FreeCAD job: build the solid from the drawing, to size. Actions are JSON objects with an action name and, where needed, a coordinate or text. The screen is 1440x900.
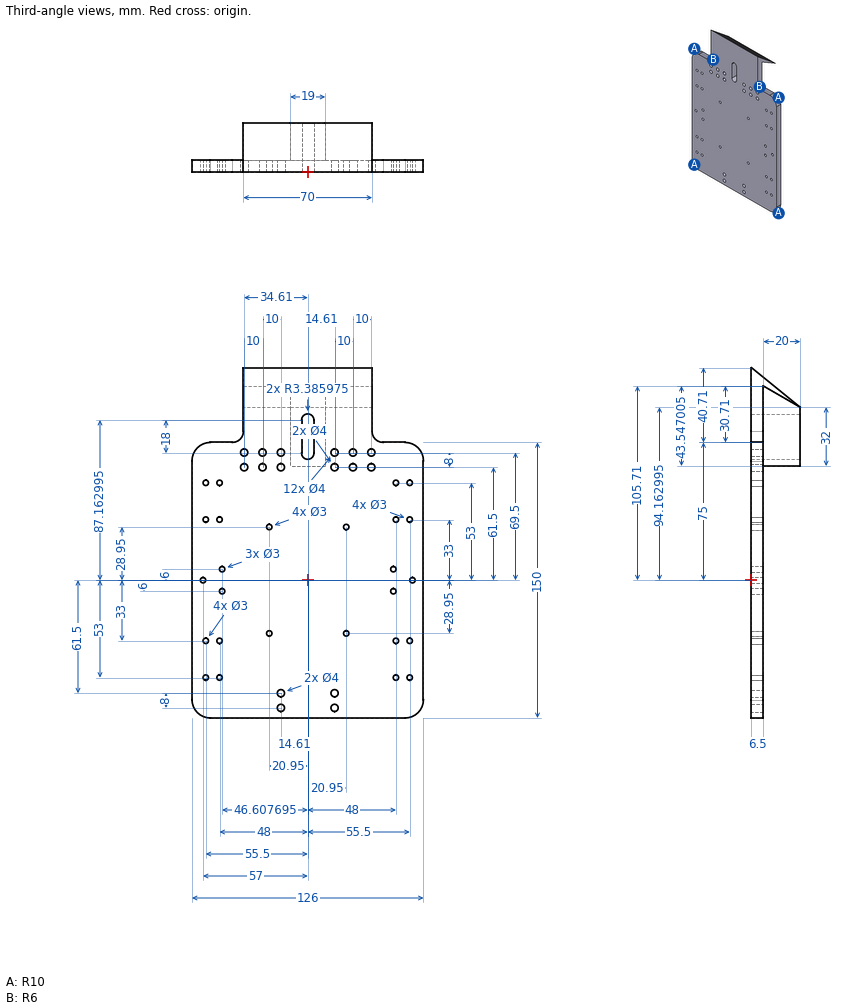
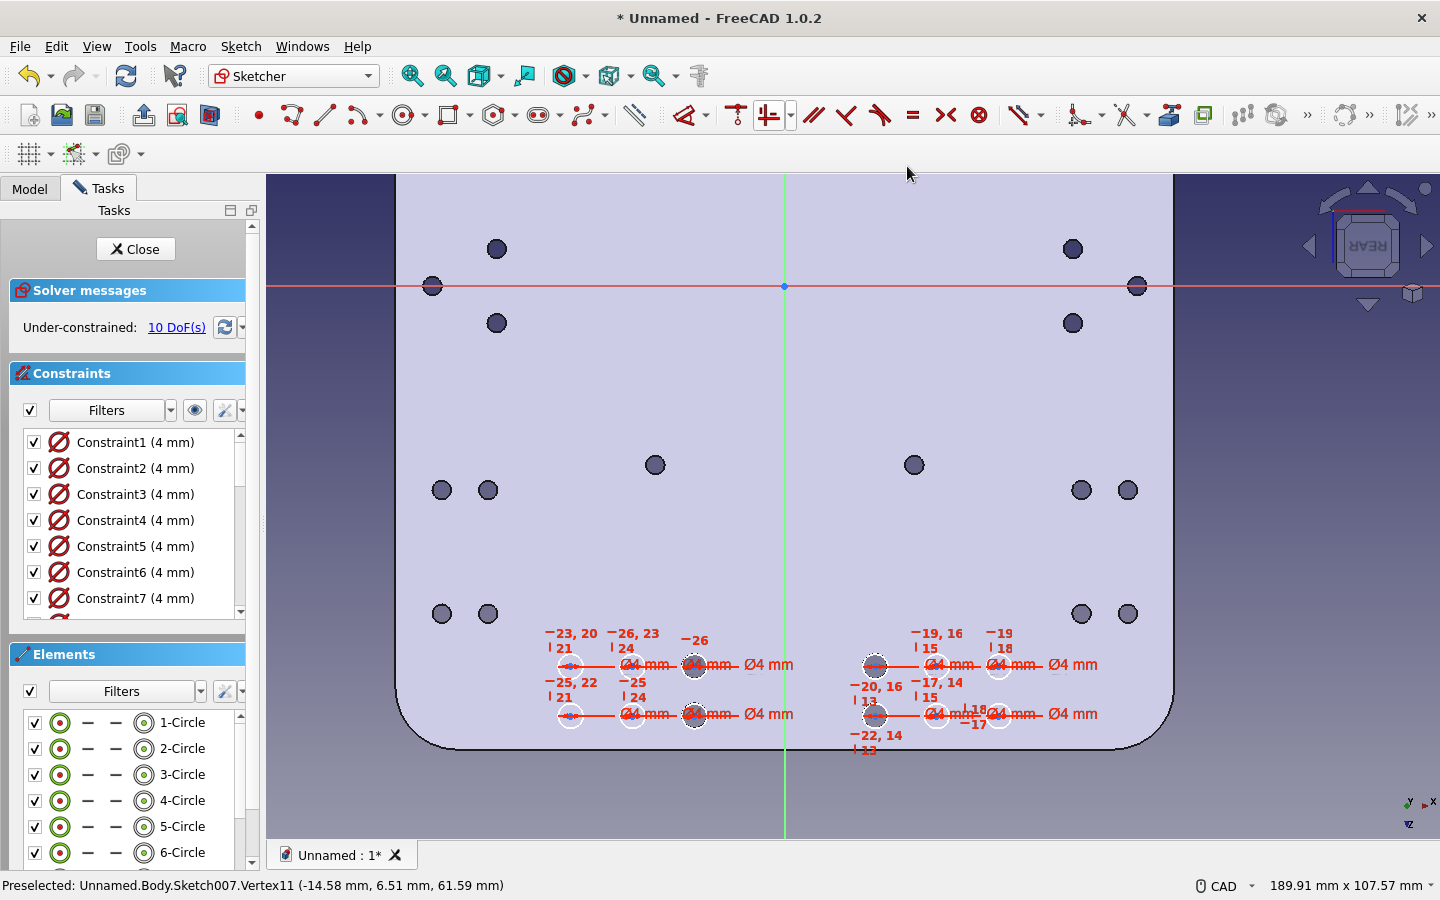
{"action": "left_click", "coordinate": [695, 667]}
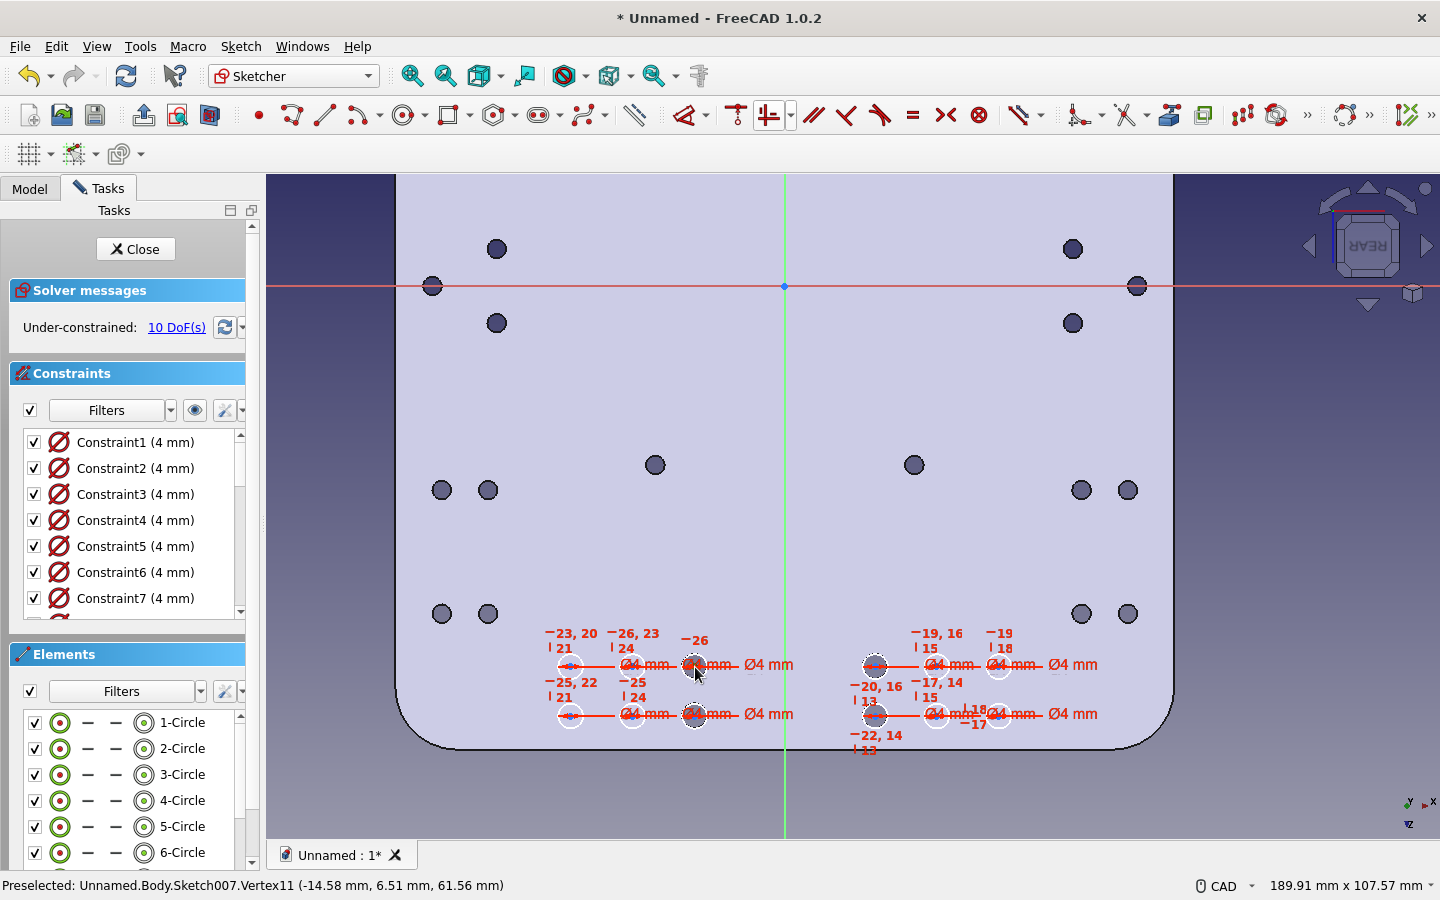
{"action": "left_click", "coordinate": [695, 716]}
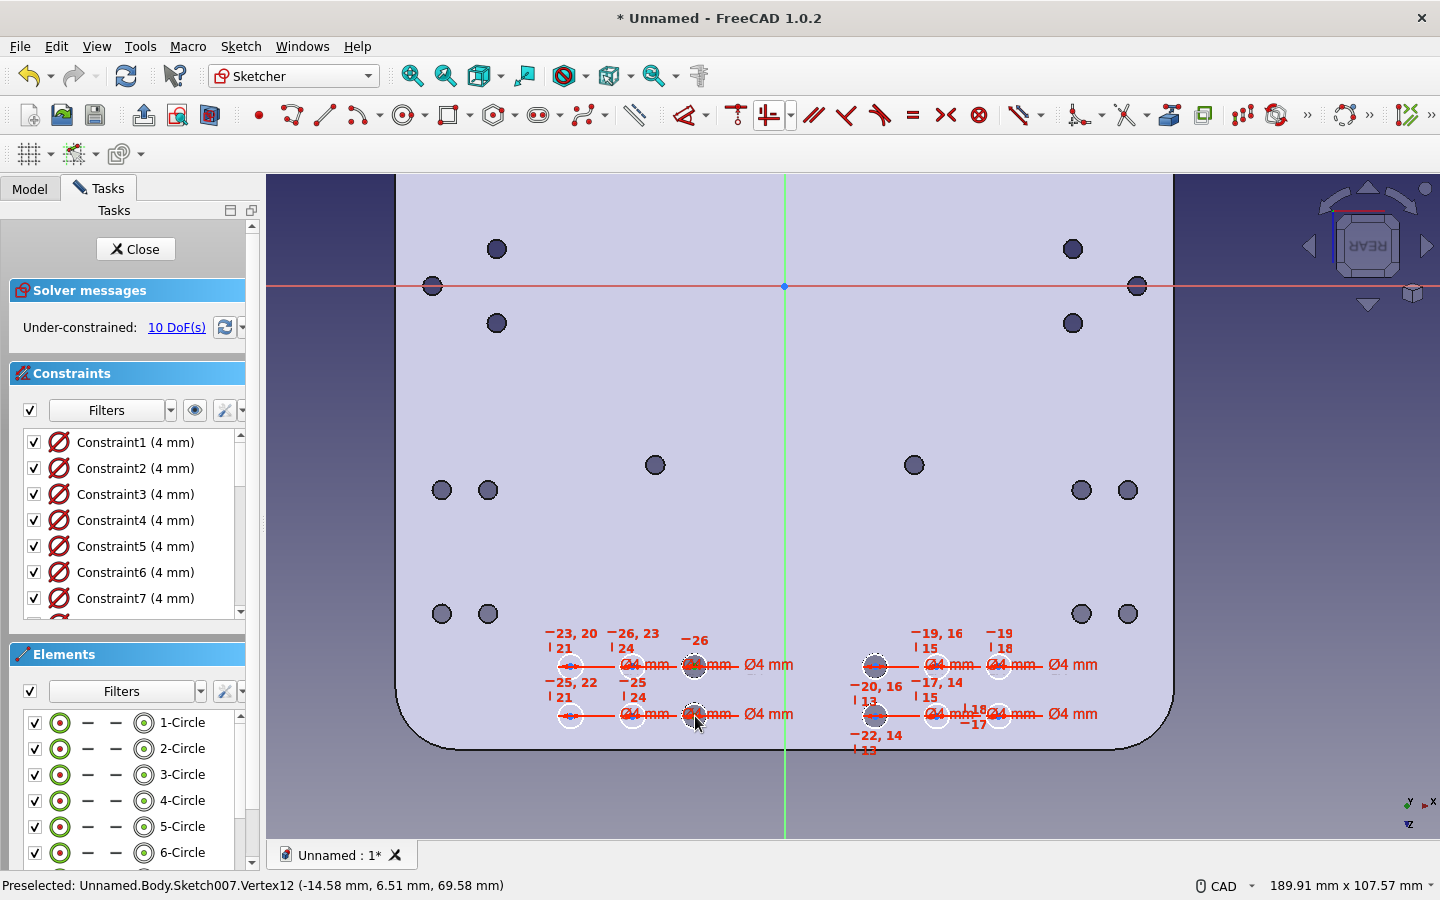
{"action": "key", "text": "v"}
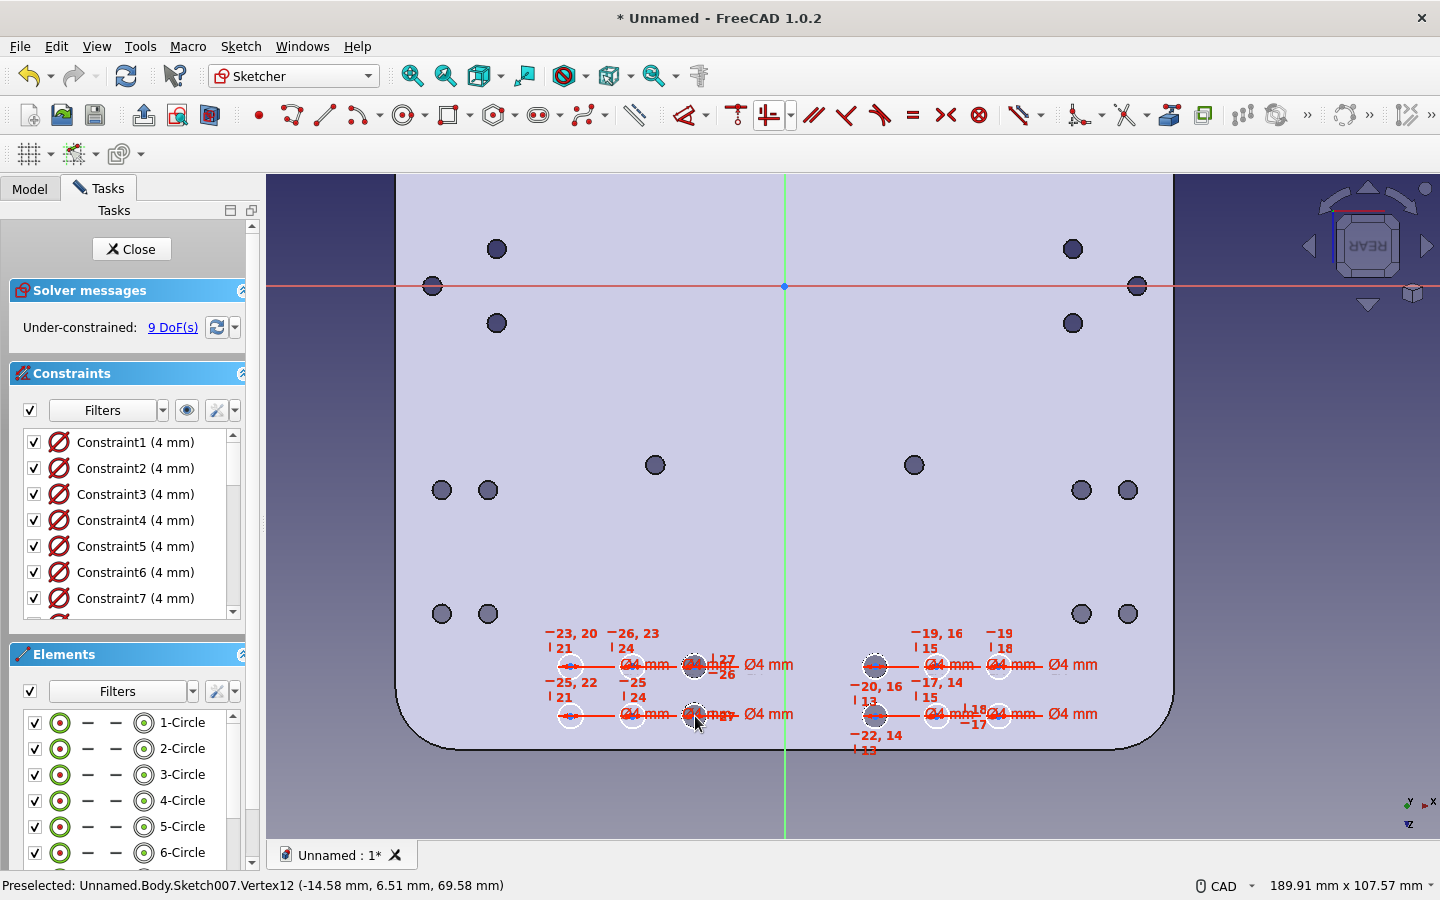
{"action": "left_click", "coordinate": [633, 716]}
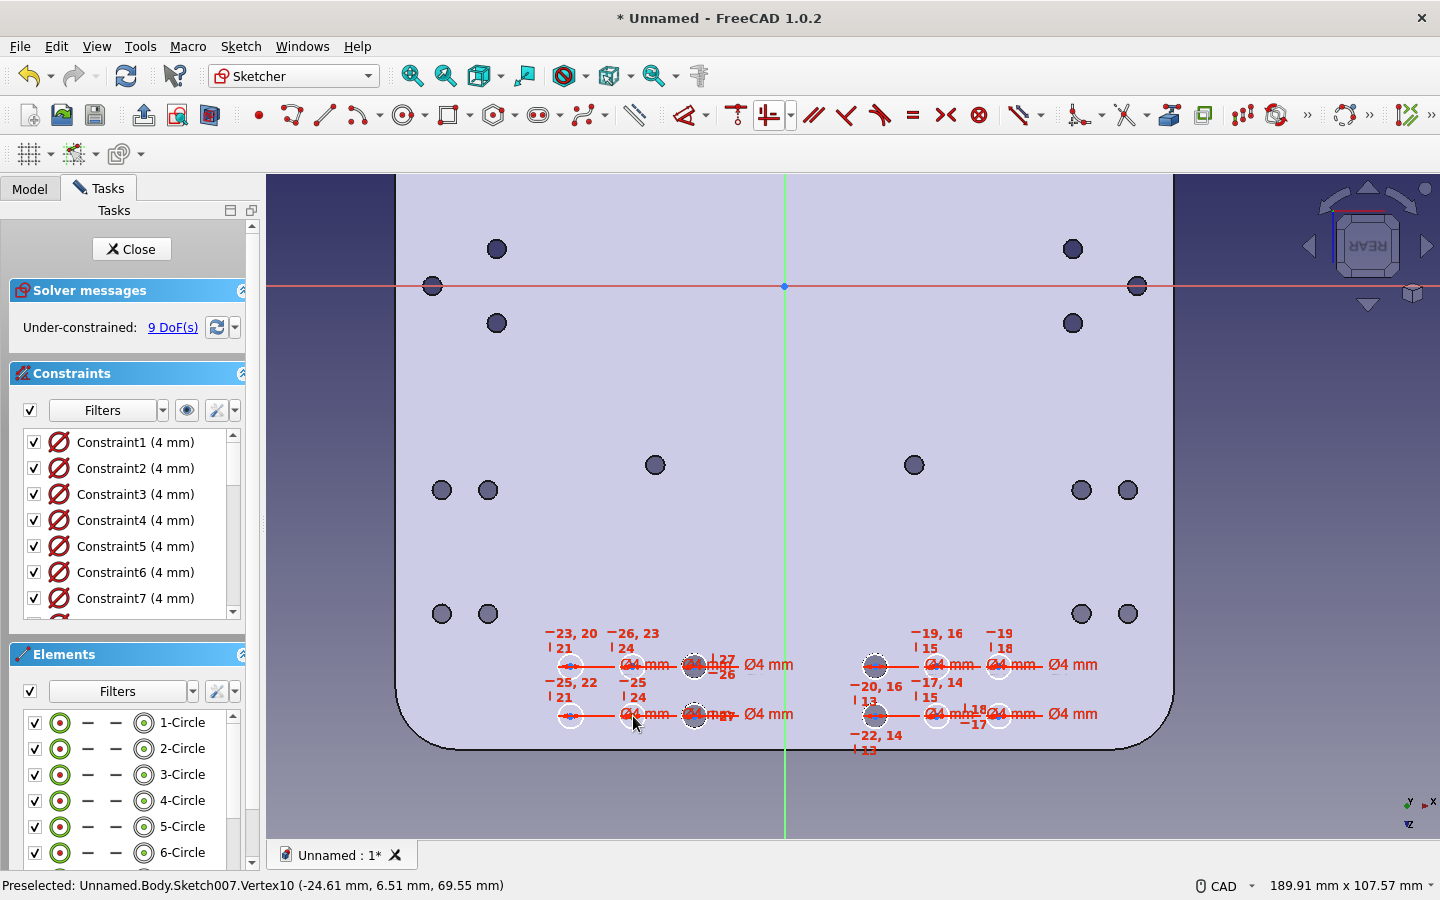
{"action": "left_click", "coordinate": [695, 716]}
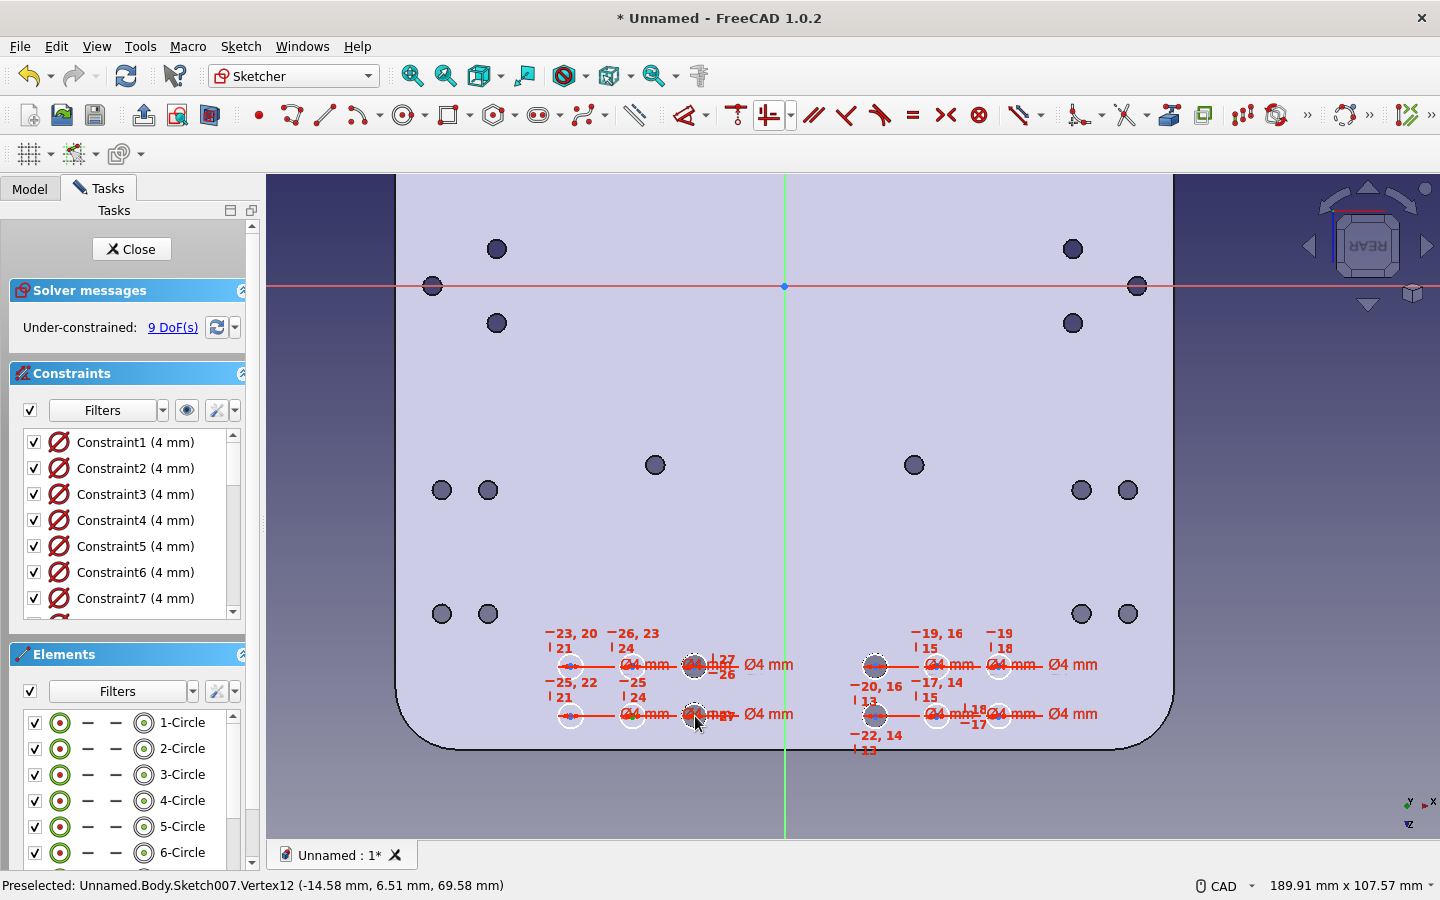
{"action": "key", "text": "h"}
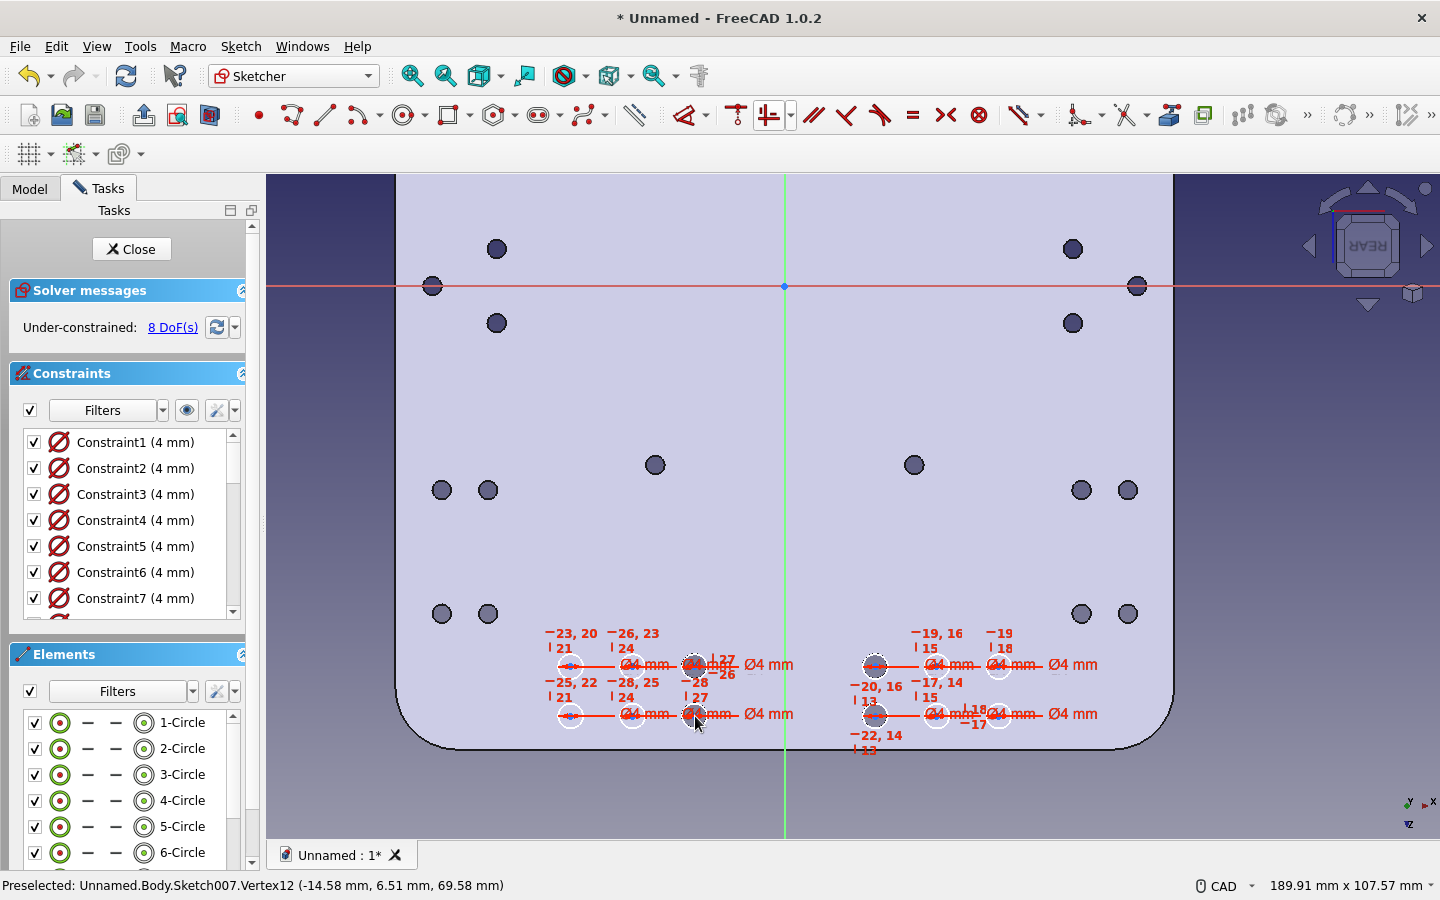
{"action": "left_click", "coordinate": [684, 116]}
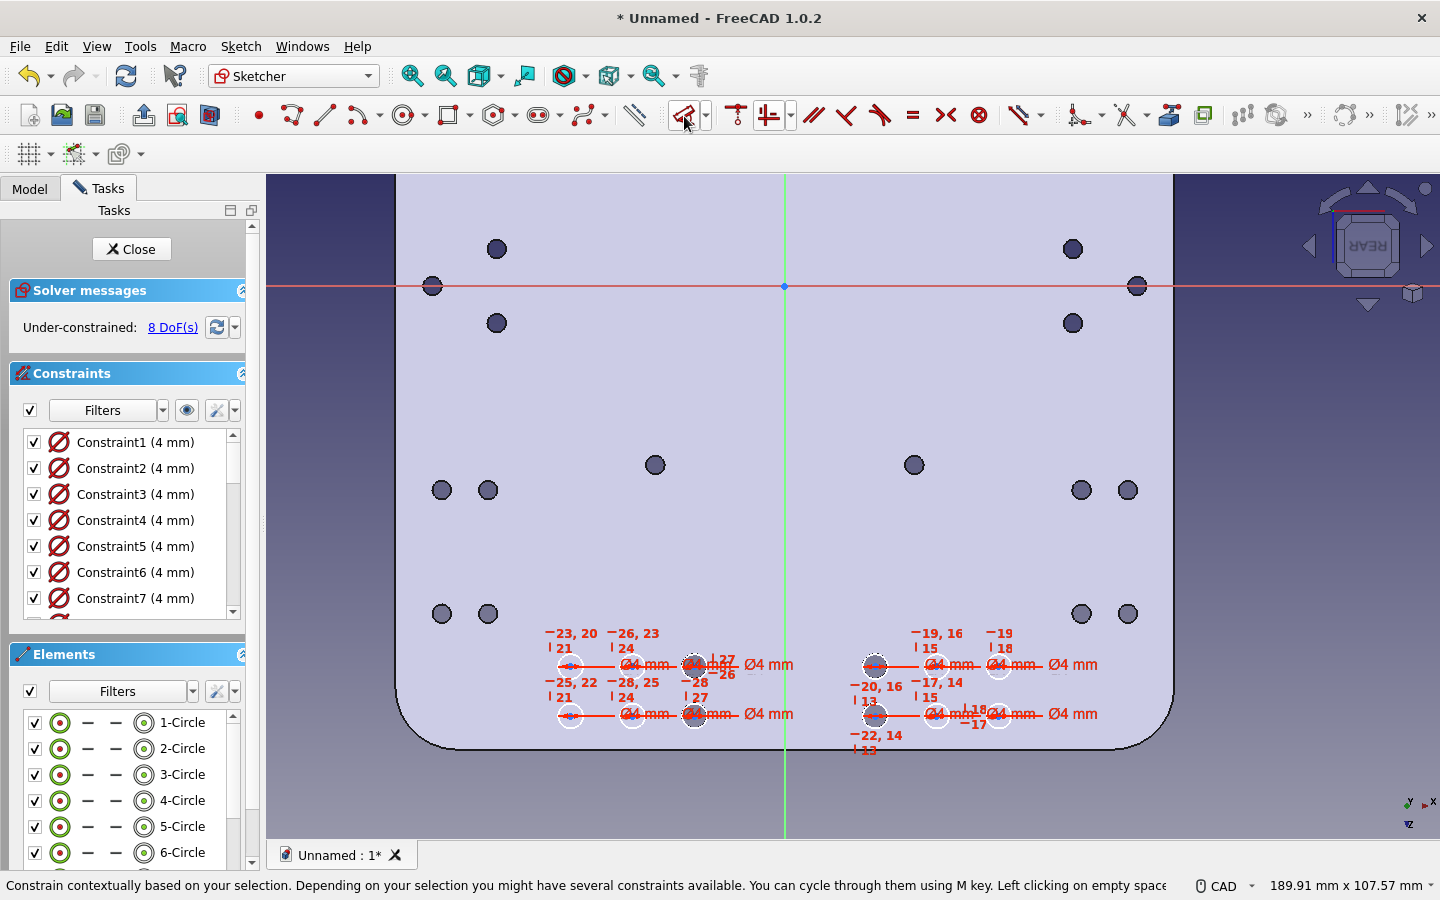
{"action": "left_click", "coordinate": [875, 716]}